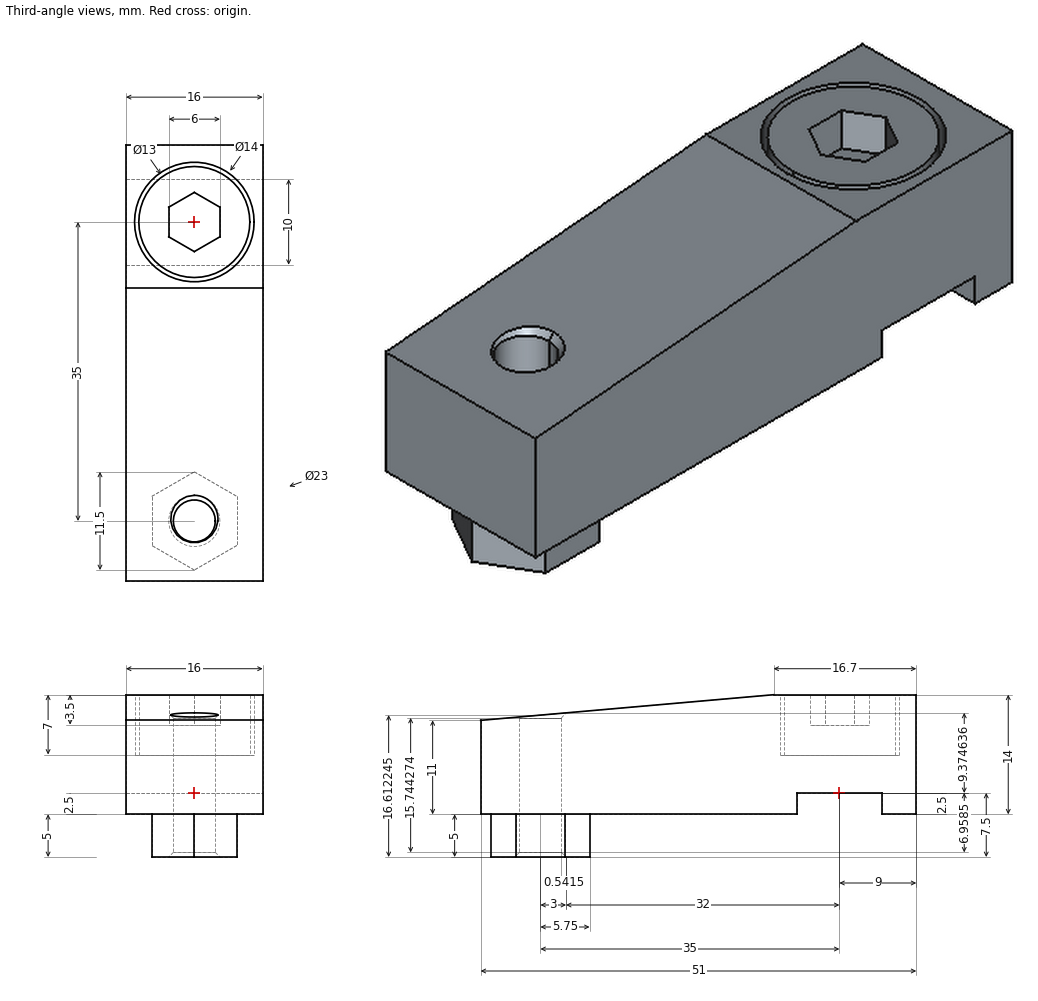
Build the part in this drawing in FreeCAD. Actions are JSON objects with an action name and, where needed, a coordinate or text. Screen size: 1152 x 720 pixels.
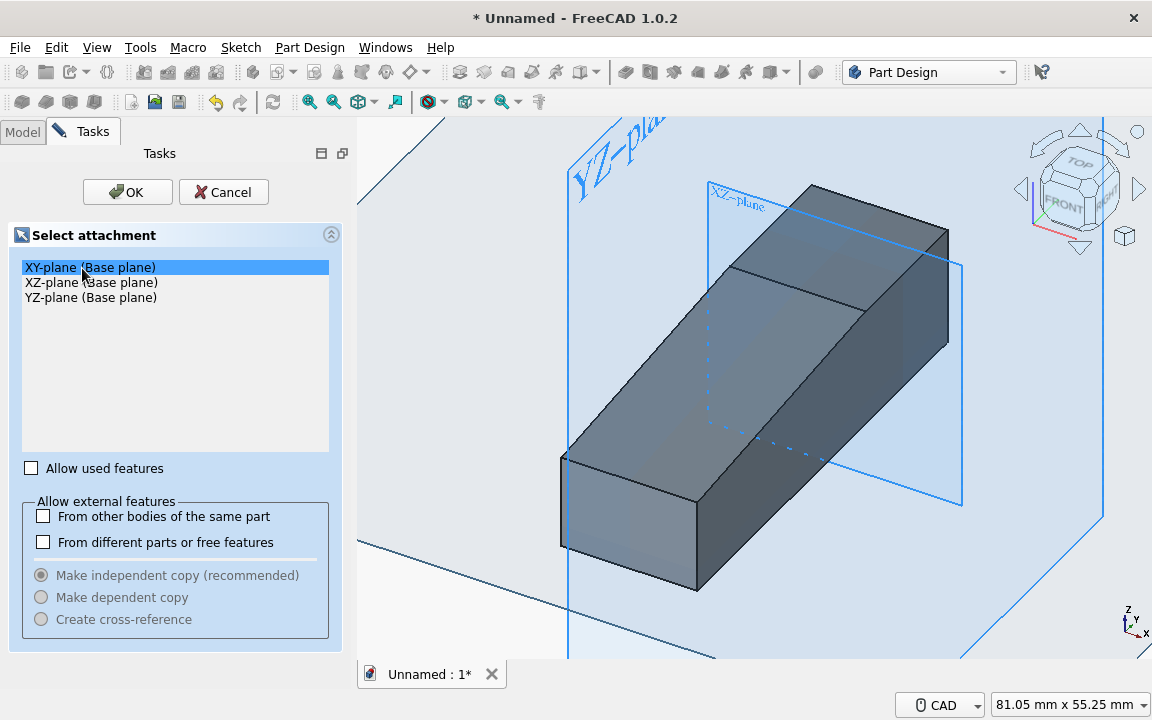
{"action": "left_click", "coordinate": [128, 192]}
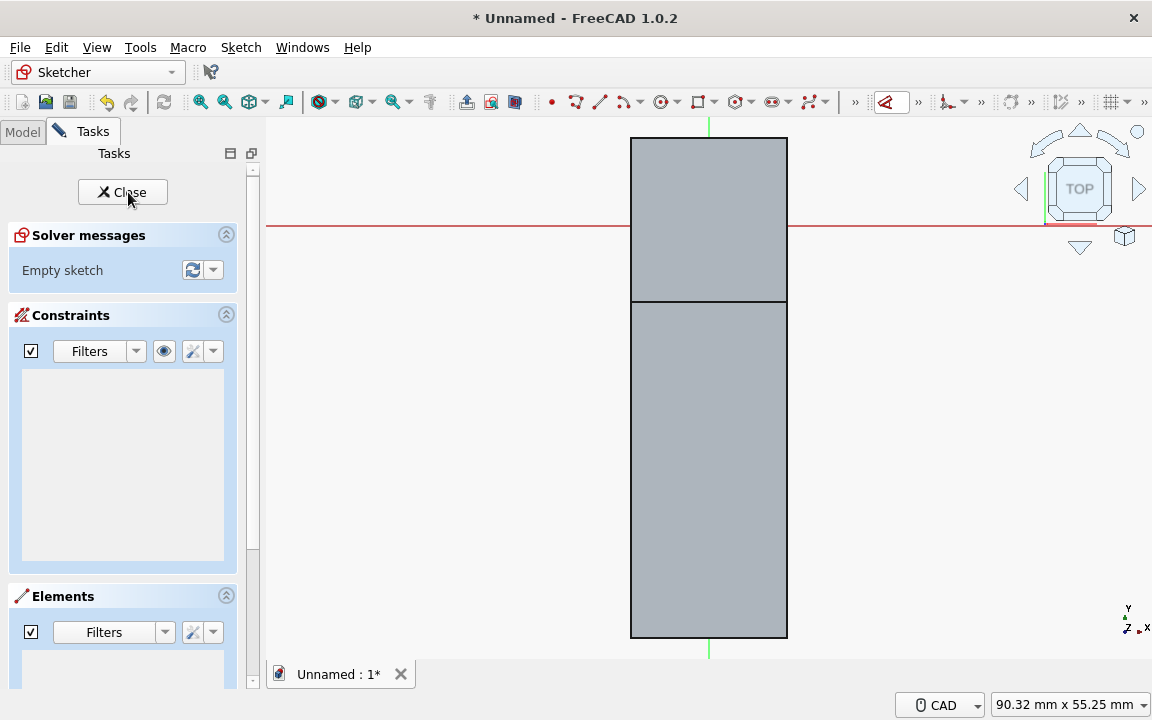
{"action": "left_click", "coordinate": [516, 102]}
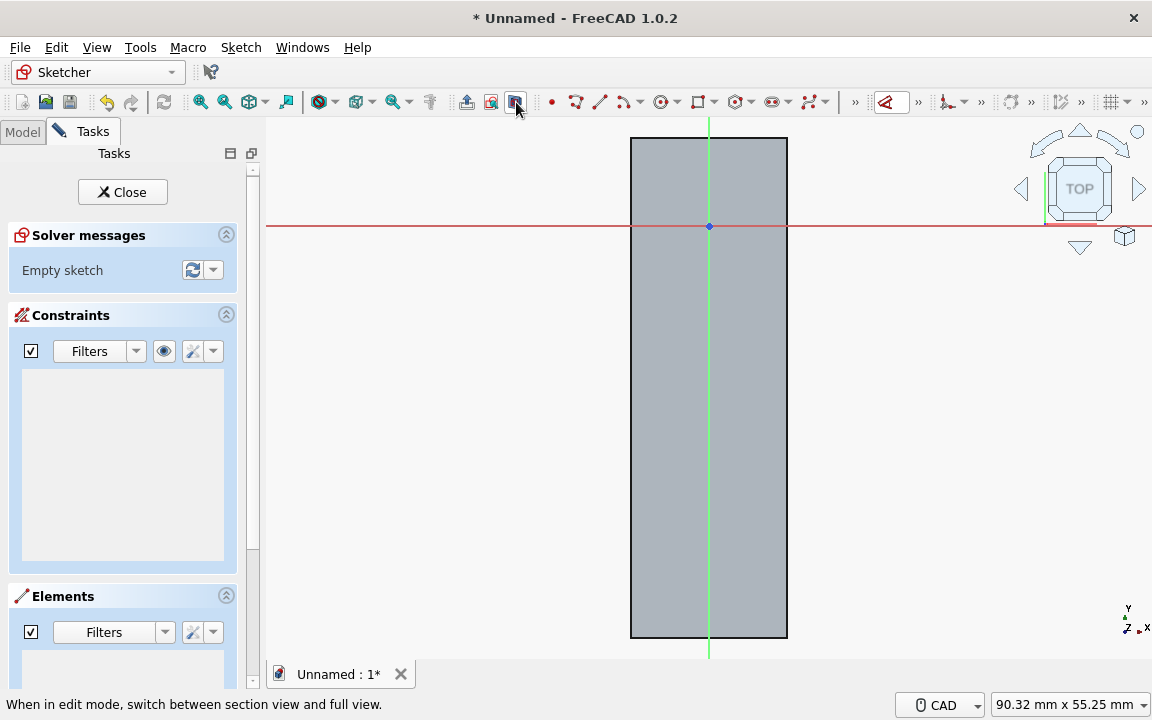
{"action": "scroll", "coordinate": [739, 156], "scroll_direction": "up", "scroll_amount": 6}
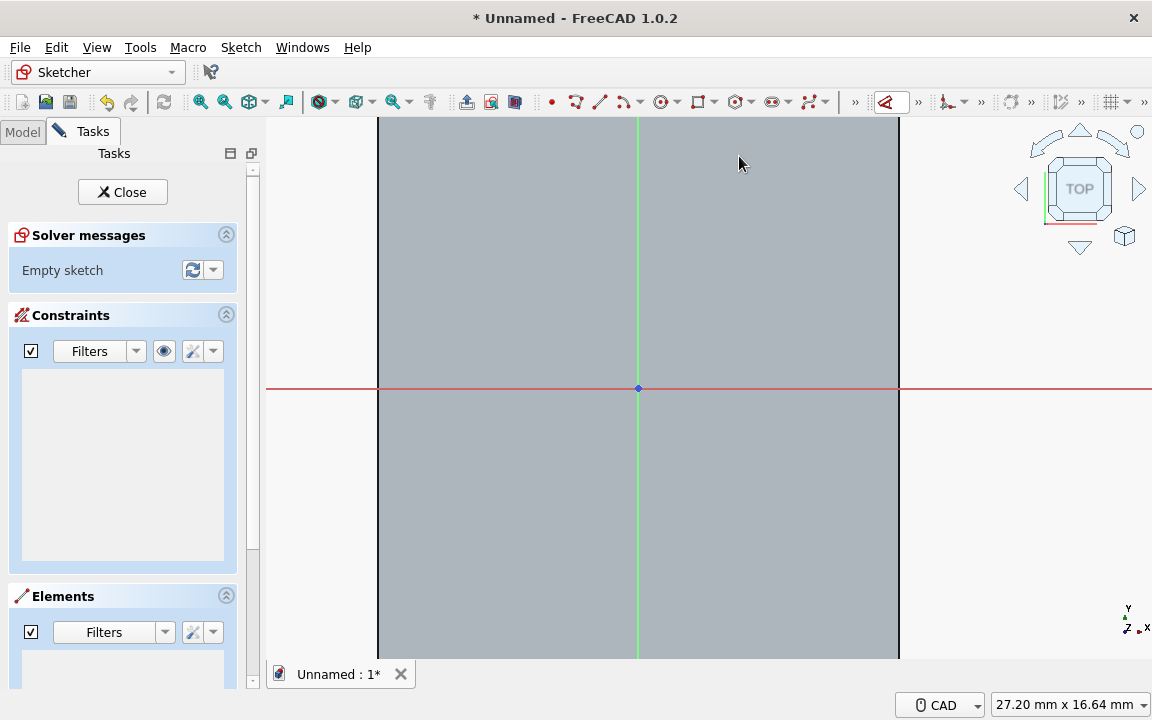
{"action": "key", "text": "g v"}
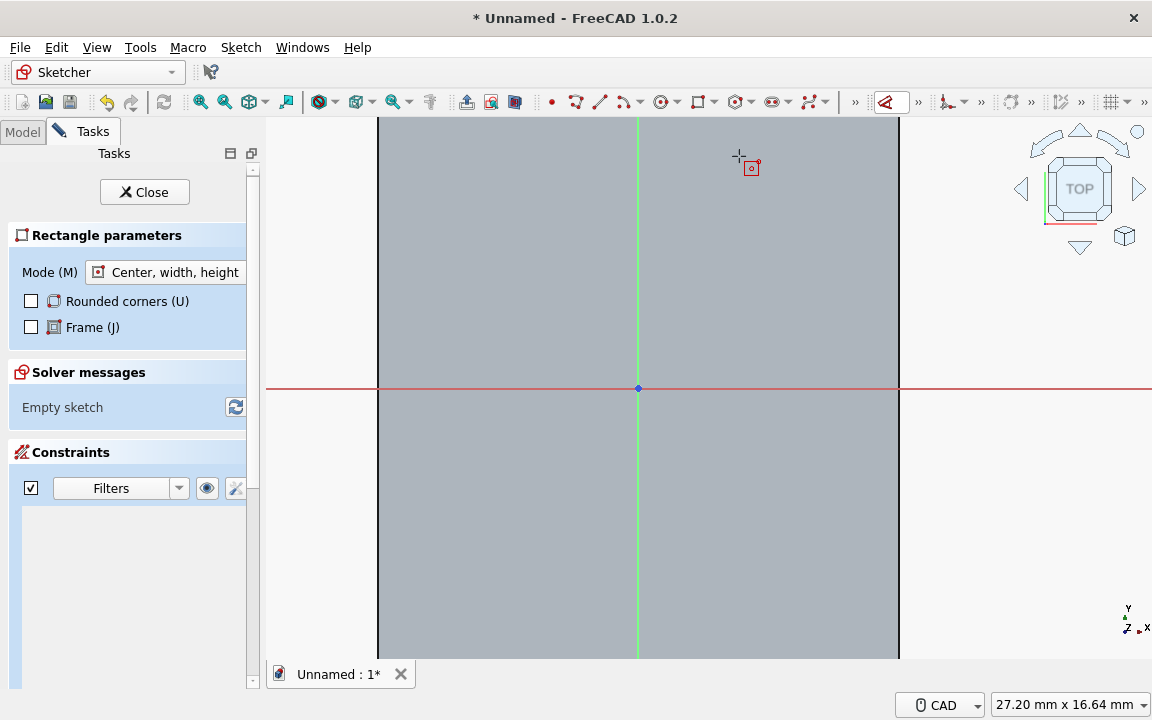
{"action": "left_click", "coordinate": [638, 389]}
{"action": "left_click", "coordinate": [899, 226]}
{"action": "key", "text": "Escape"}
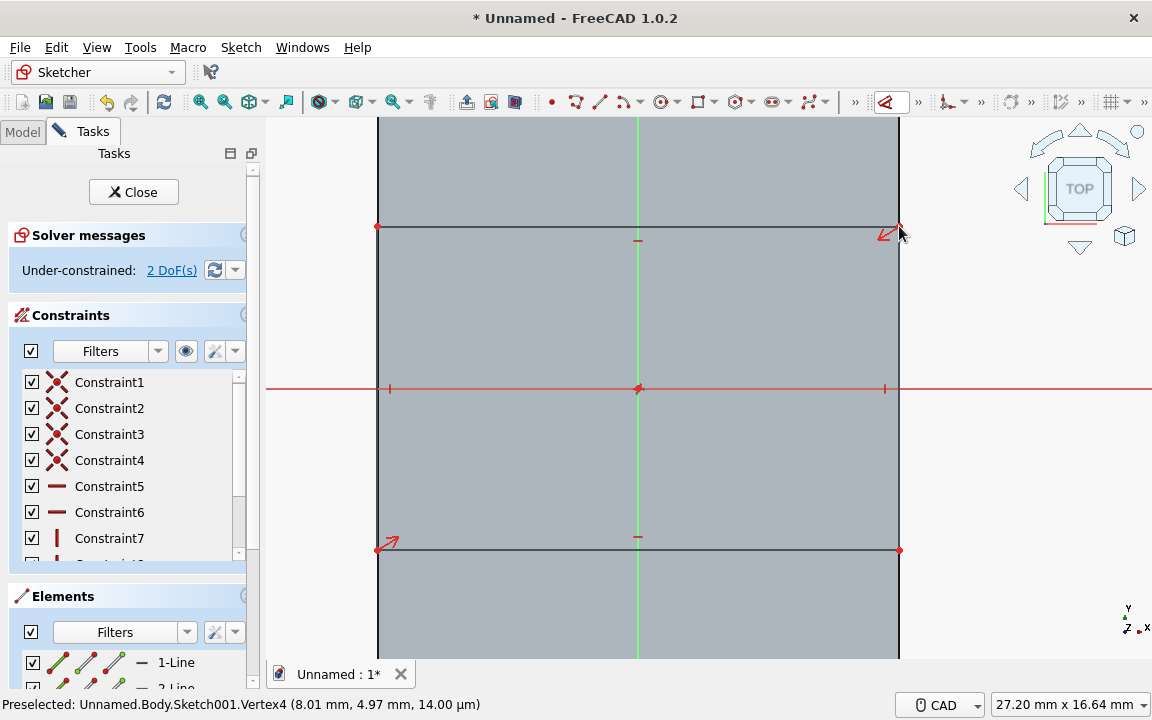
{"action": "left_click", "coordinate": [534, 550]}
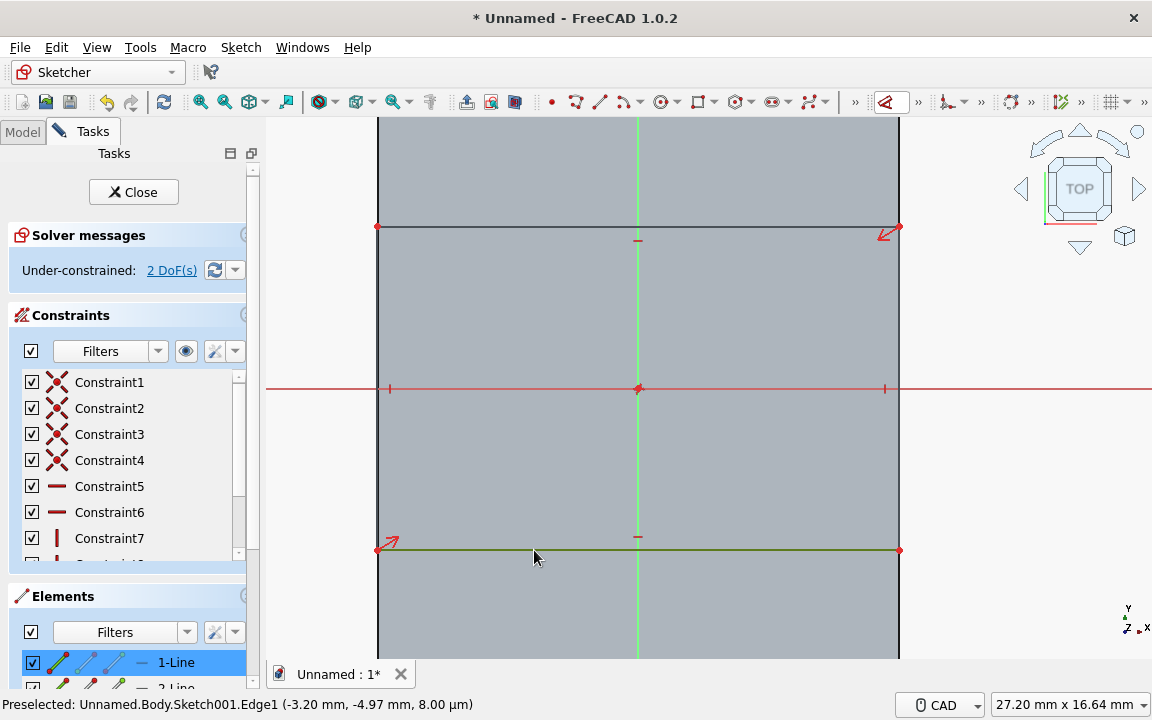
{"action": "key", "text": "l"}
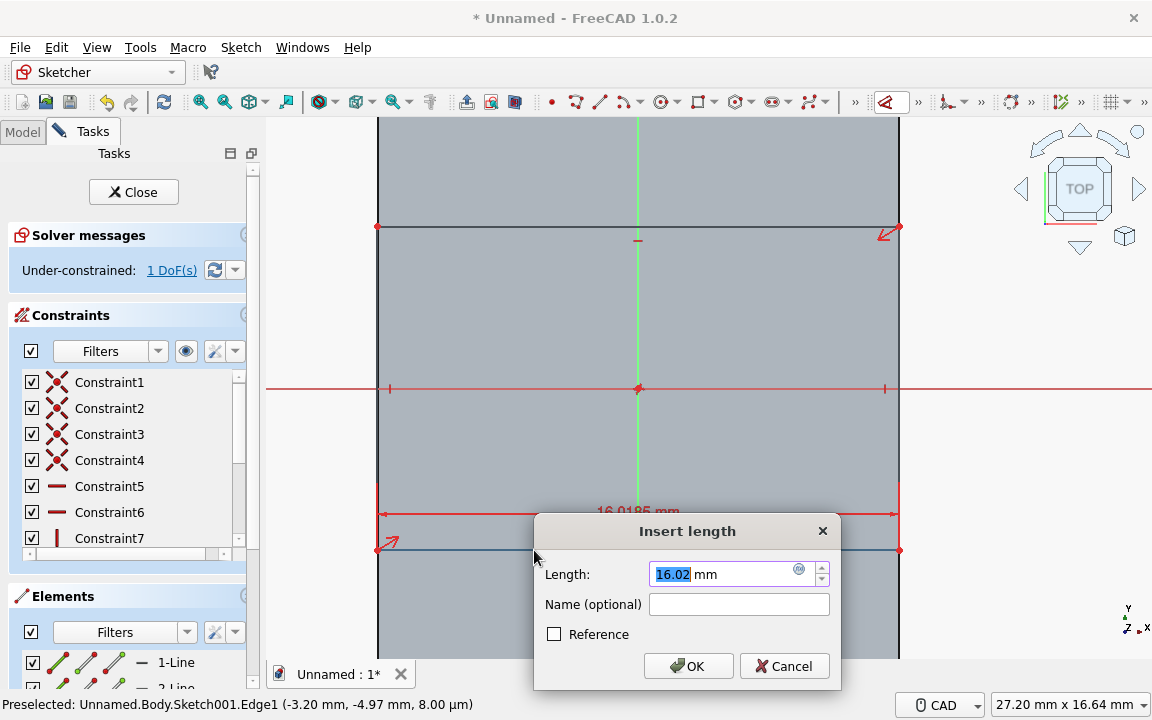
{"action": "type", "text": "16"}
{"action": "key", "text": "Return"}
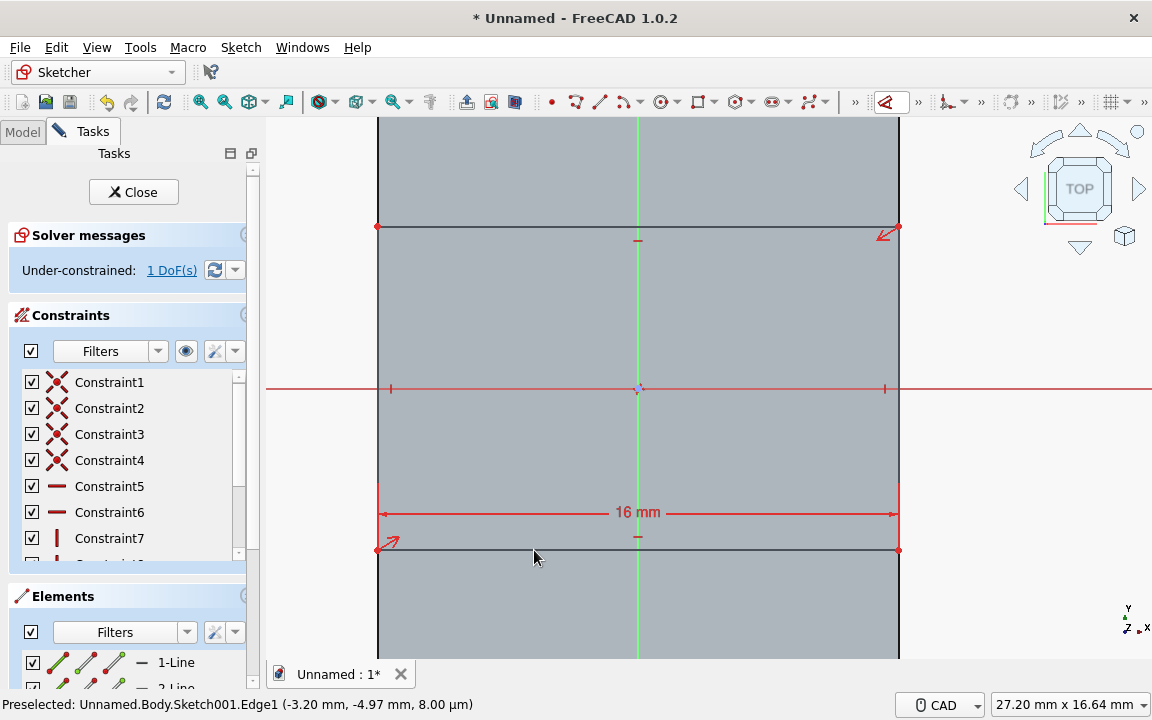
{"action": "left_click", "coordinate": [899, 453]}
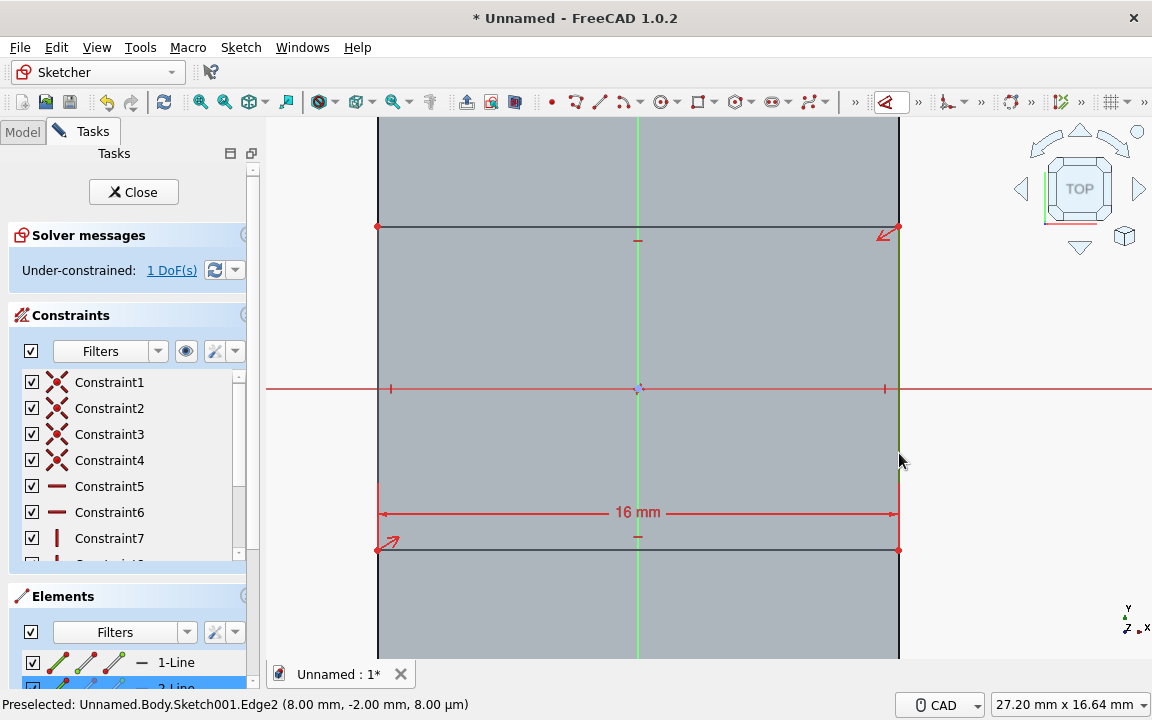
{"action": "left_click", "coordinate": [904, 102]}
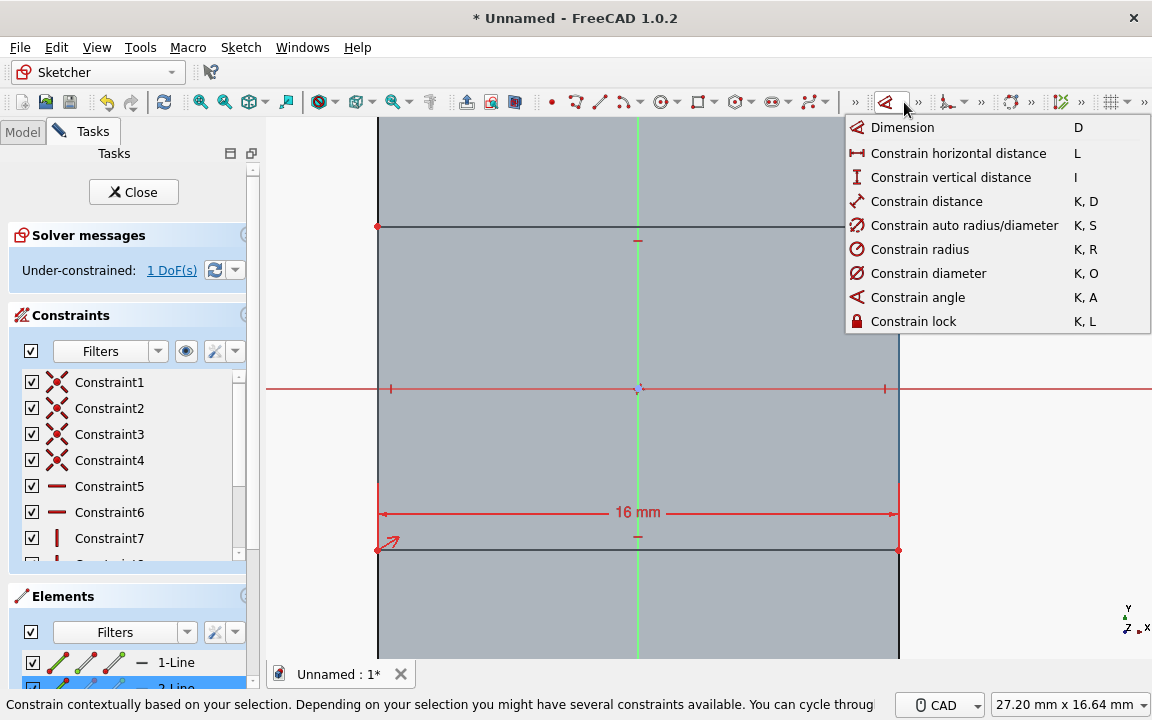
{"action": "left_click", "coordinate": [998, 177]}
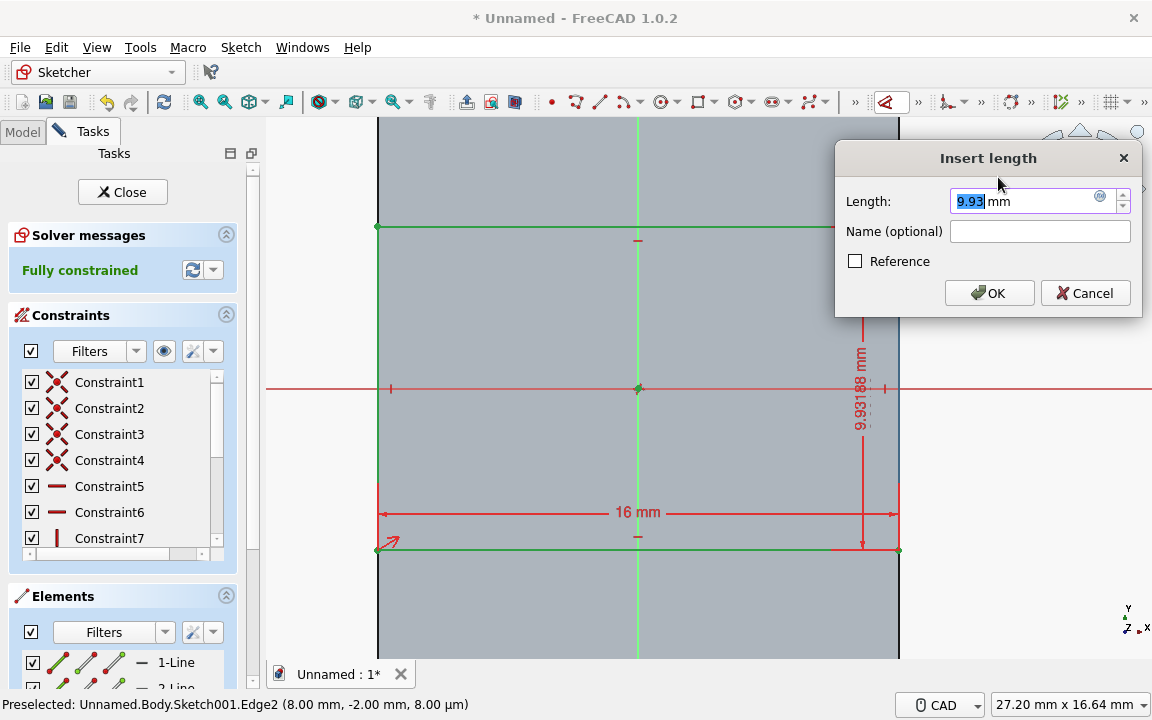
{"action": "type", "text": "10"}
{"action": "key", "text": "Return"}